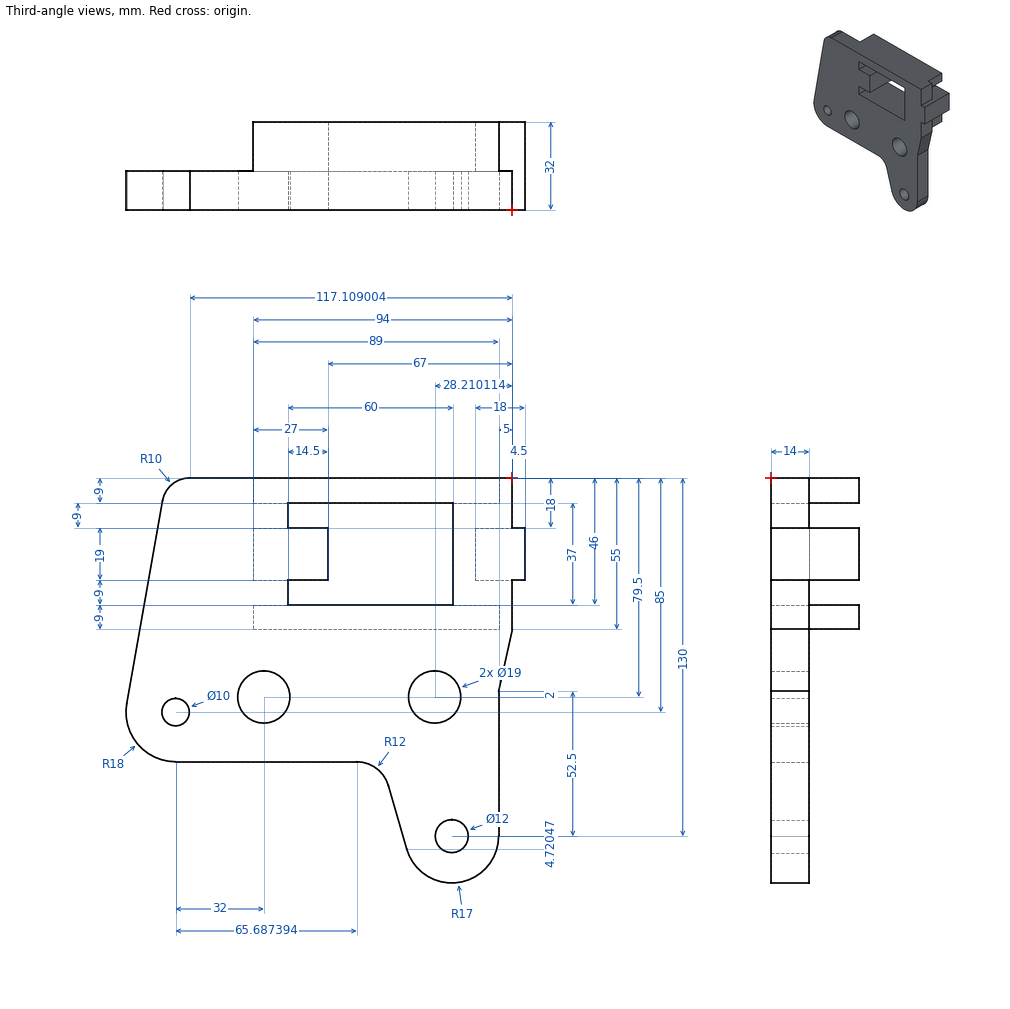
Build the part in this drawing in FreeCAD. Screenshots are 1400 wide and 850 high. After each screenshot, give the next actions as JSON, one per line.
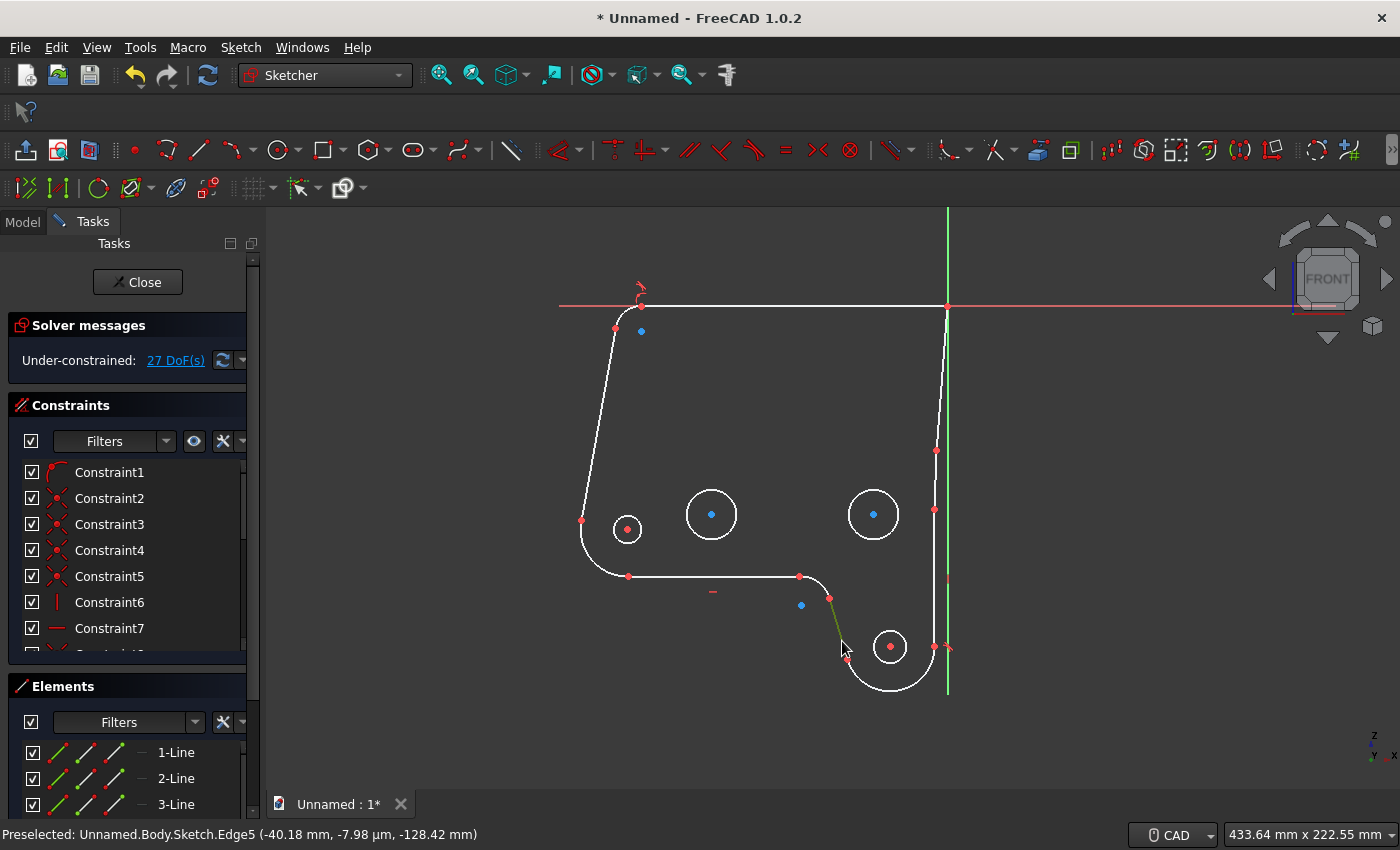
{"action": "left_click", "coordinate": [872, 687]}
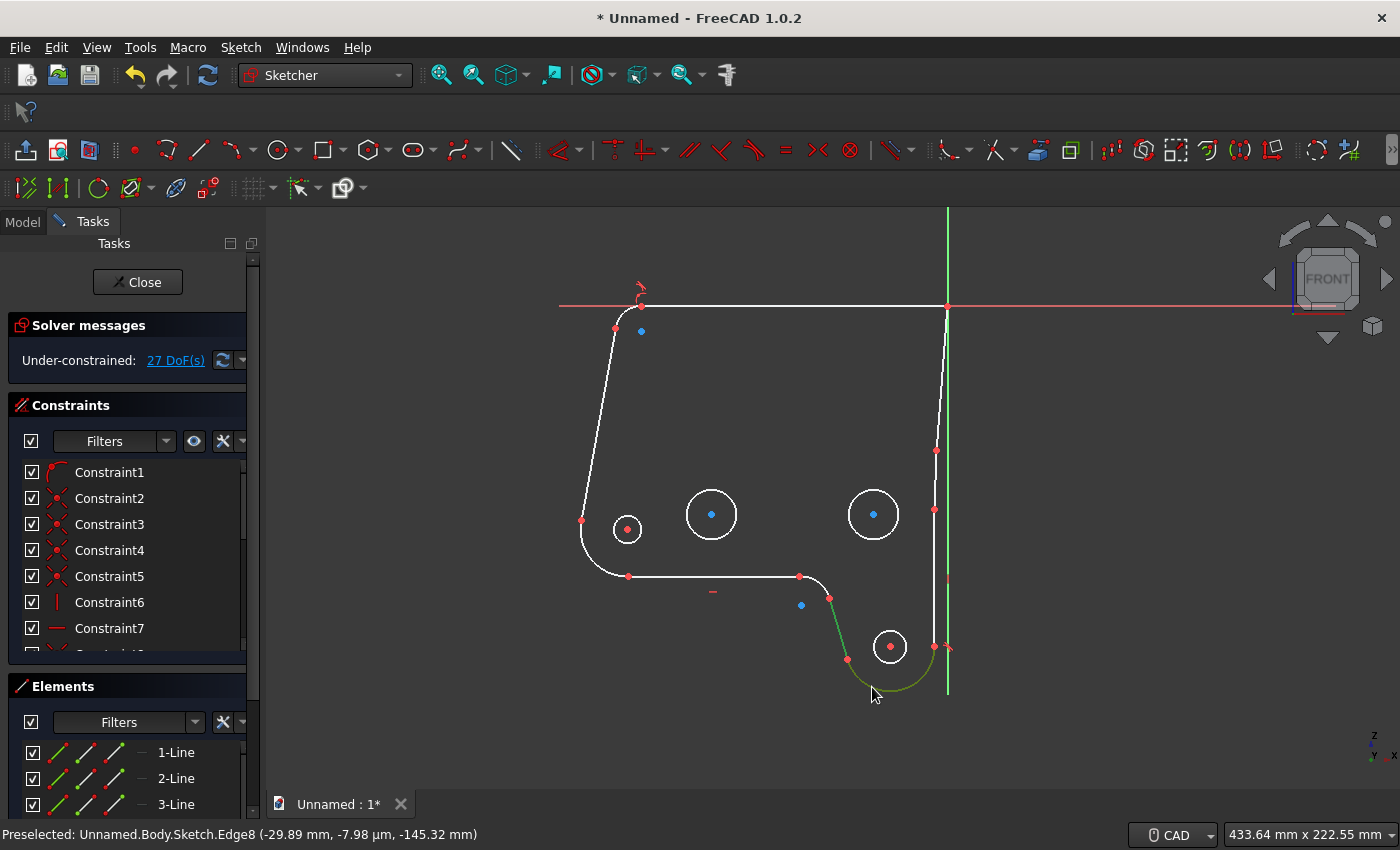
{"action": "left_click", "coordinate": [754, 150]}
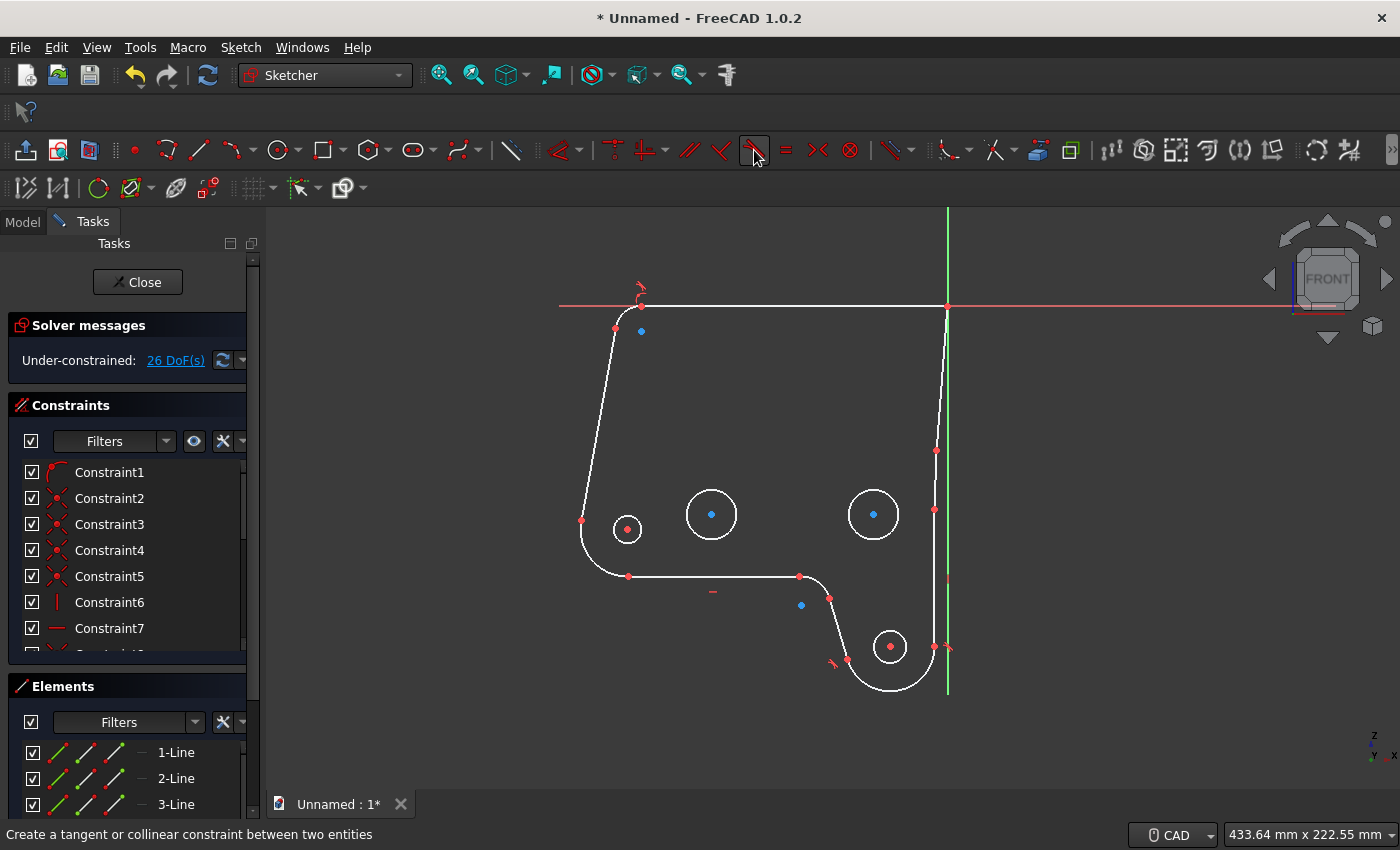
{"action": "left_click", "coordinate": [842, 641]}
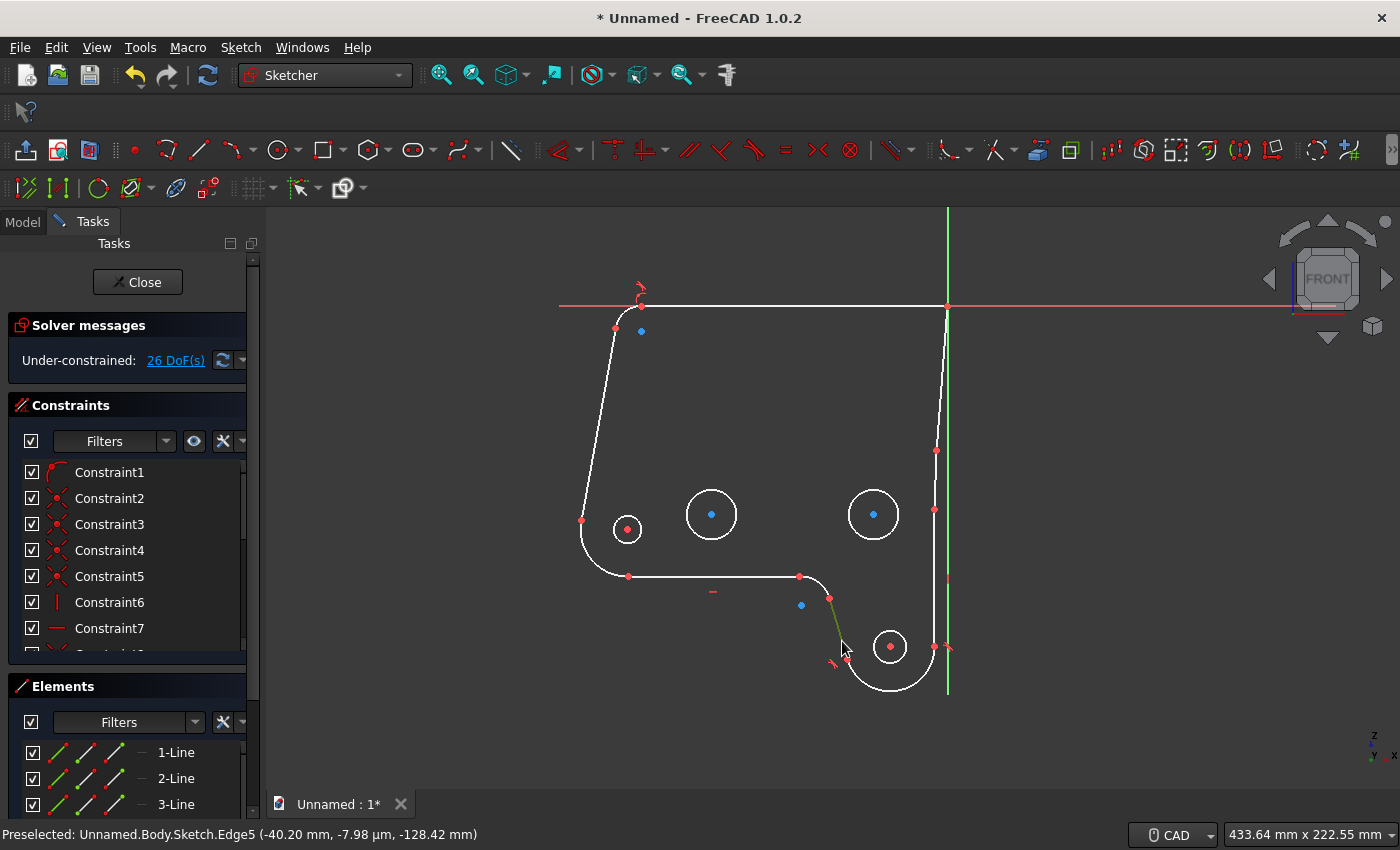
{"action": "left_click", "coordinate": [824, 588]}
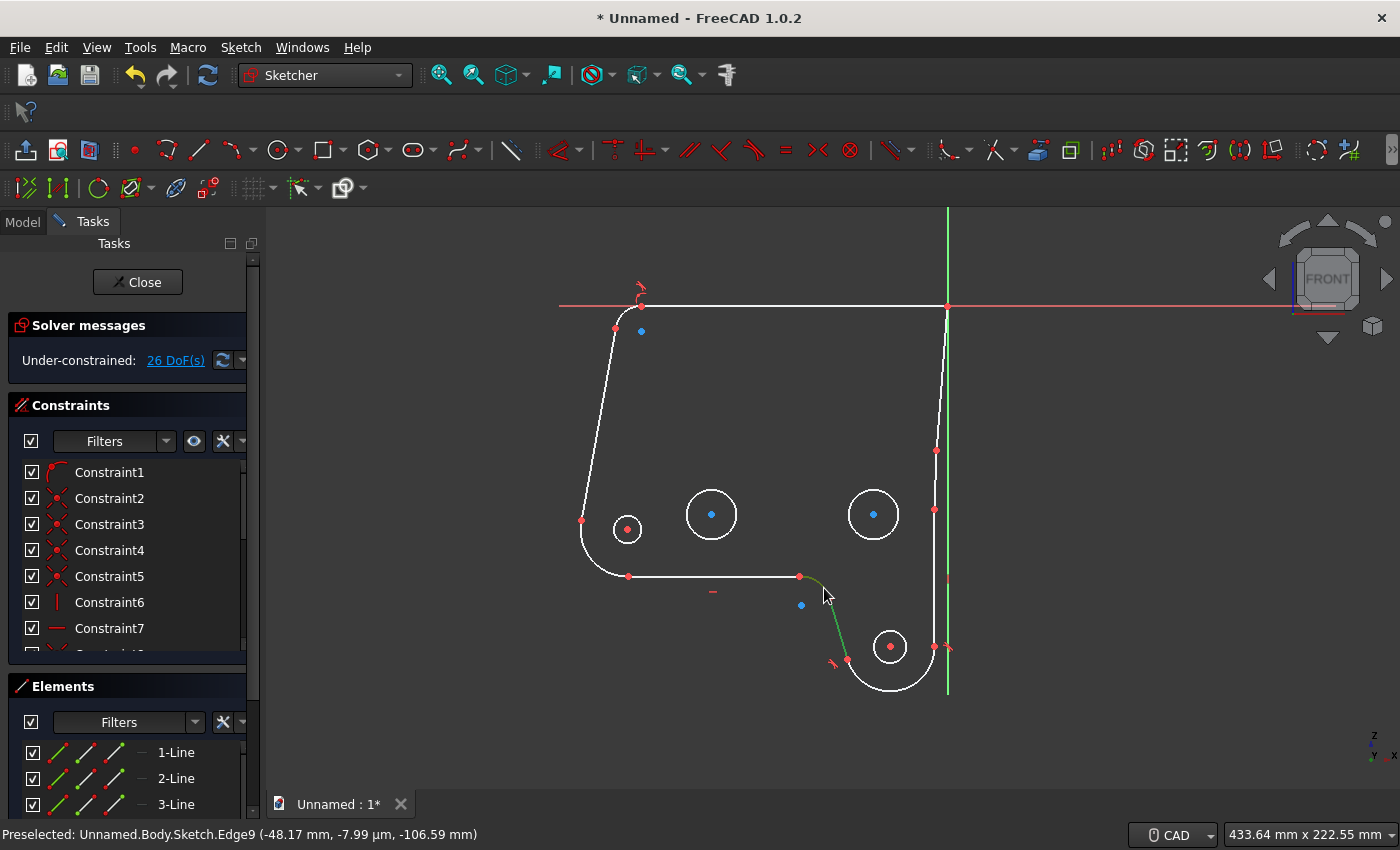
{"action": "key", "text": "t"}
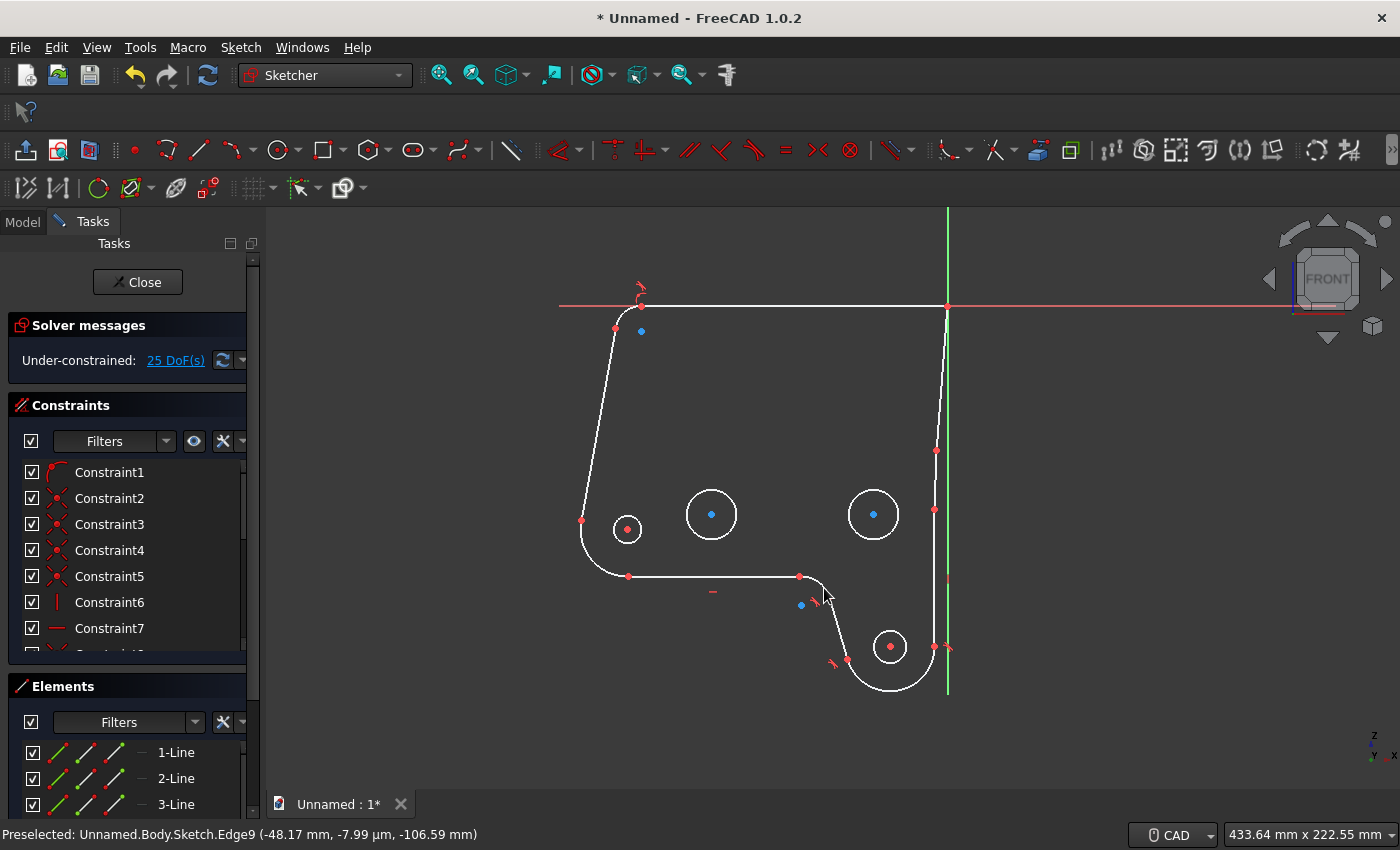
{"action": "left_click", "coordinate": [748, 577]}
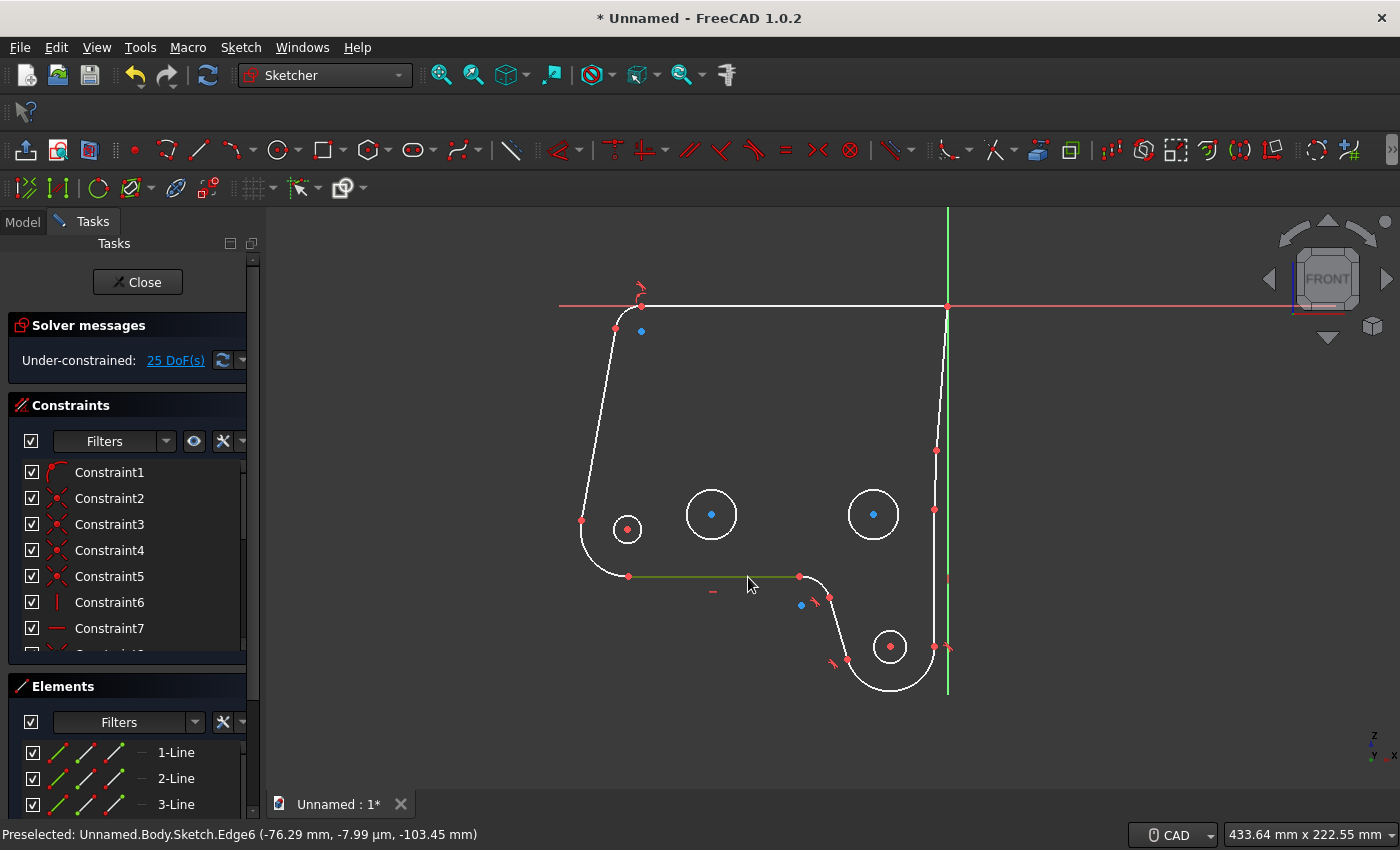
{"action": "left_click", "coordinate": [824, 587]}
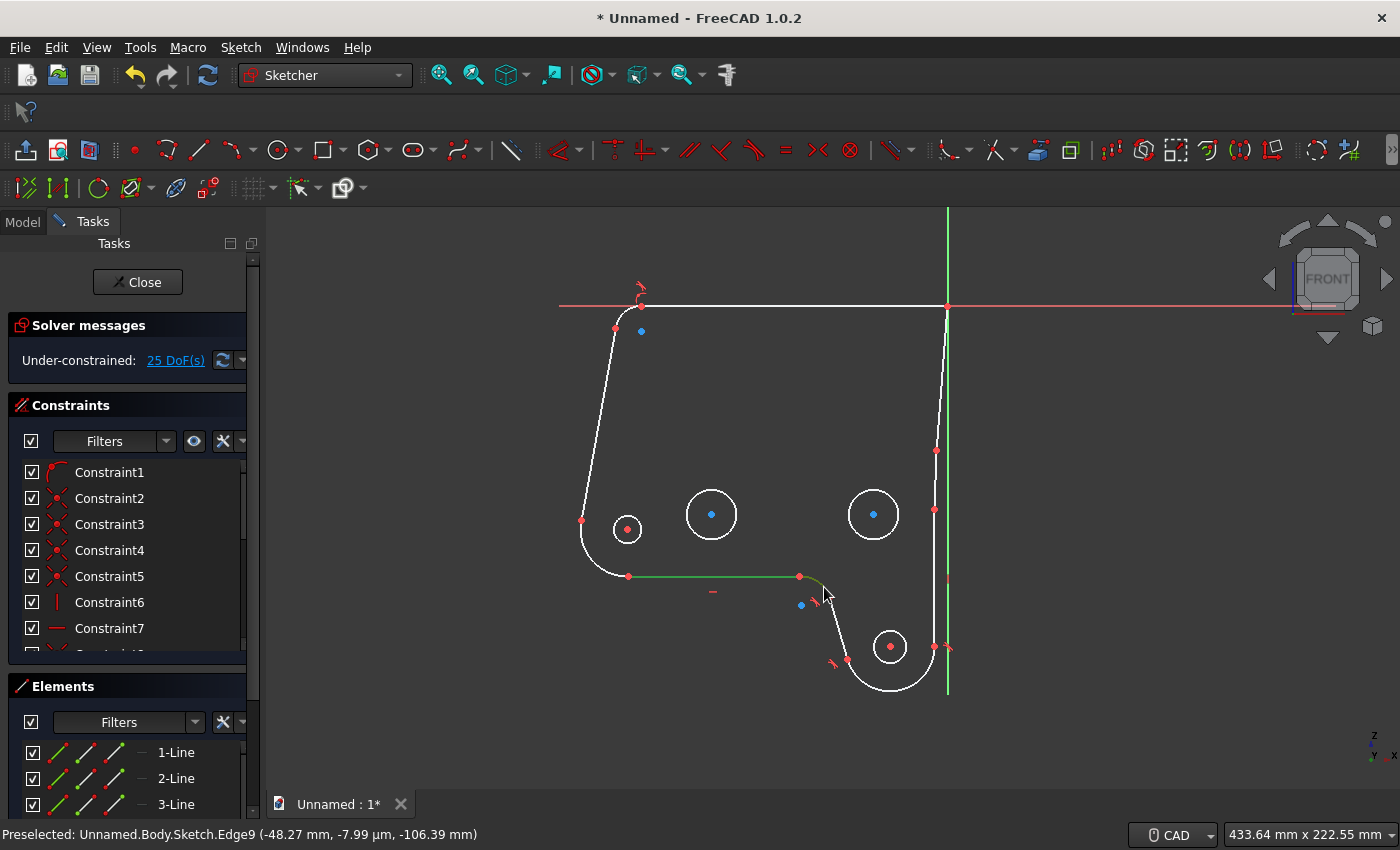
{"action": "left_click", "coordinate": [754, 150]}